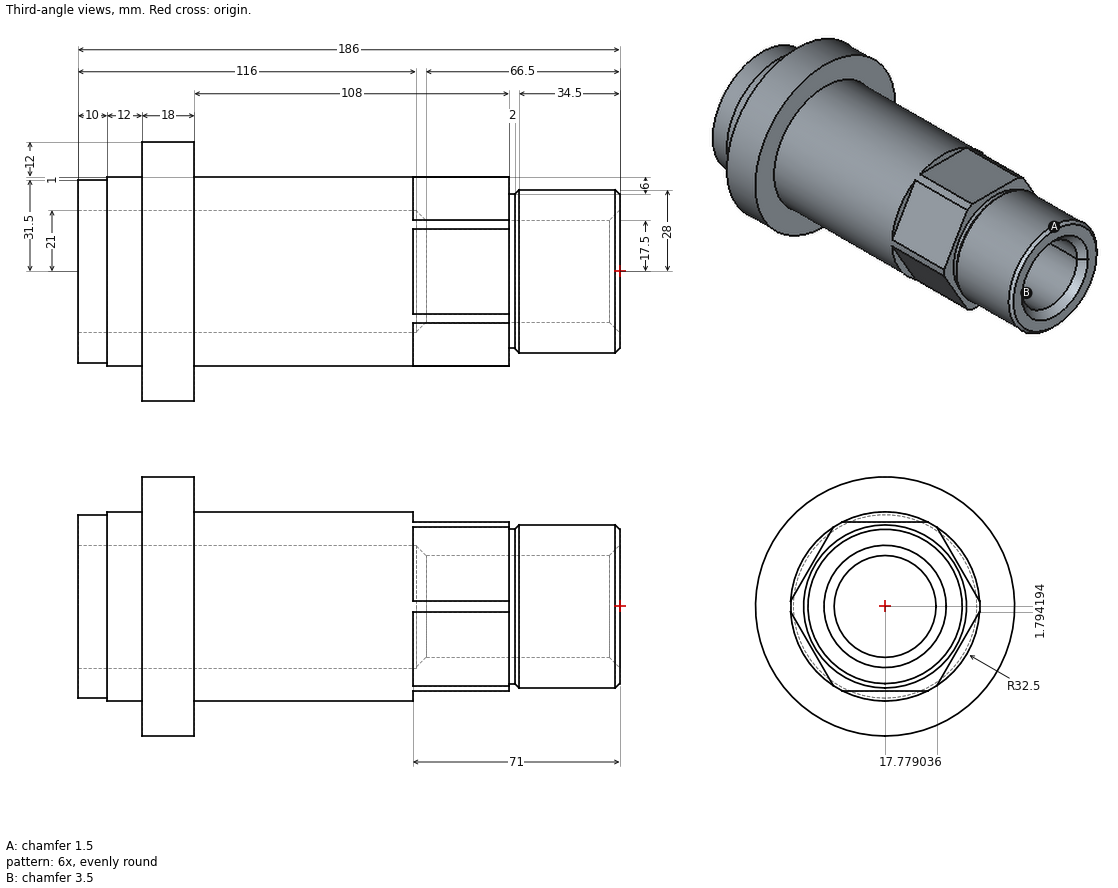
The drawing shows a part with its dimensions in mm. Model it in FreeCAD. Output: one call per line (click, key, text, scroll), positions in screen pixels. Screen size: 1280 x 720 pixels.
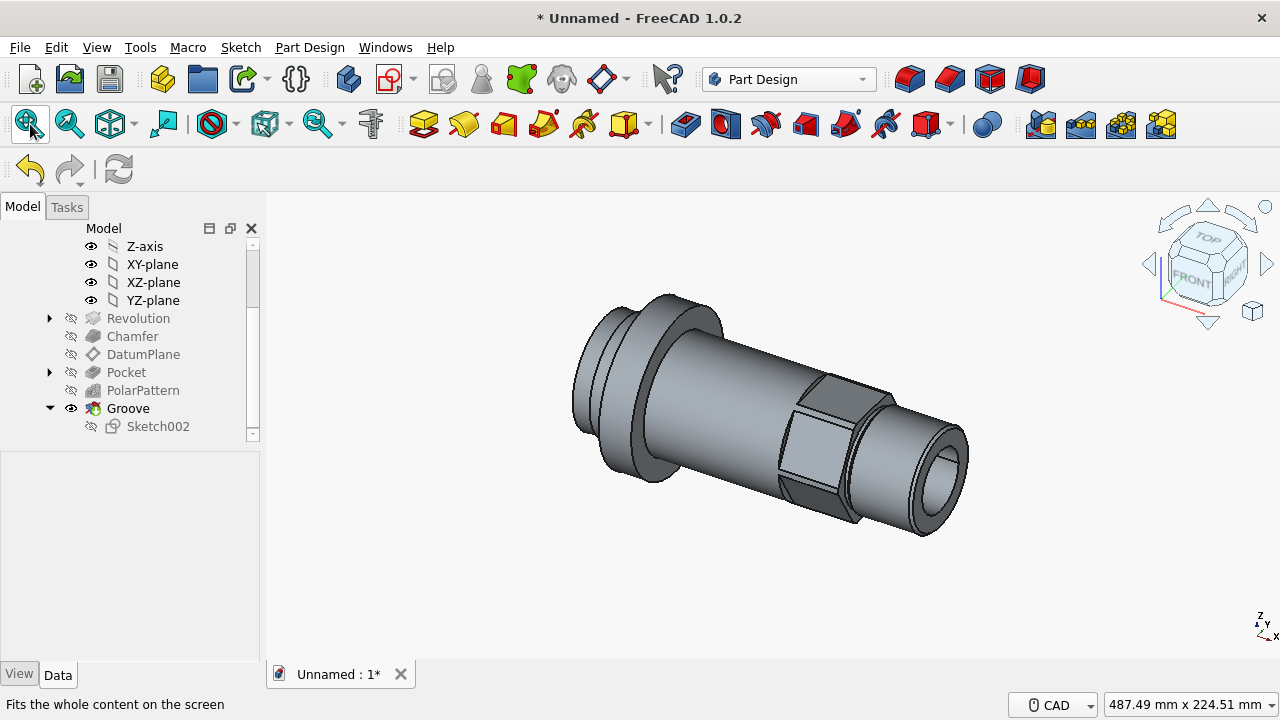
click(935, 514)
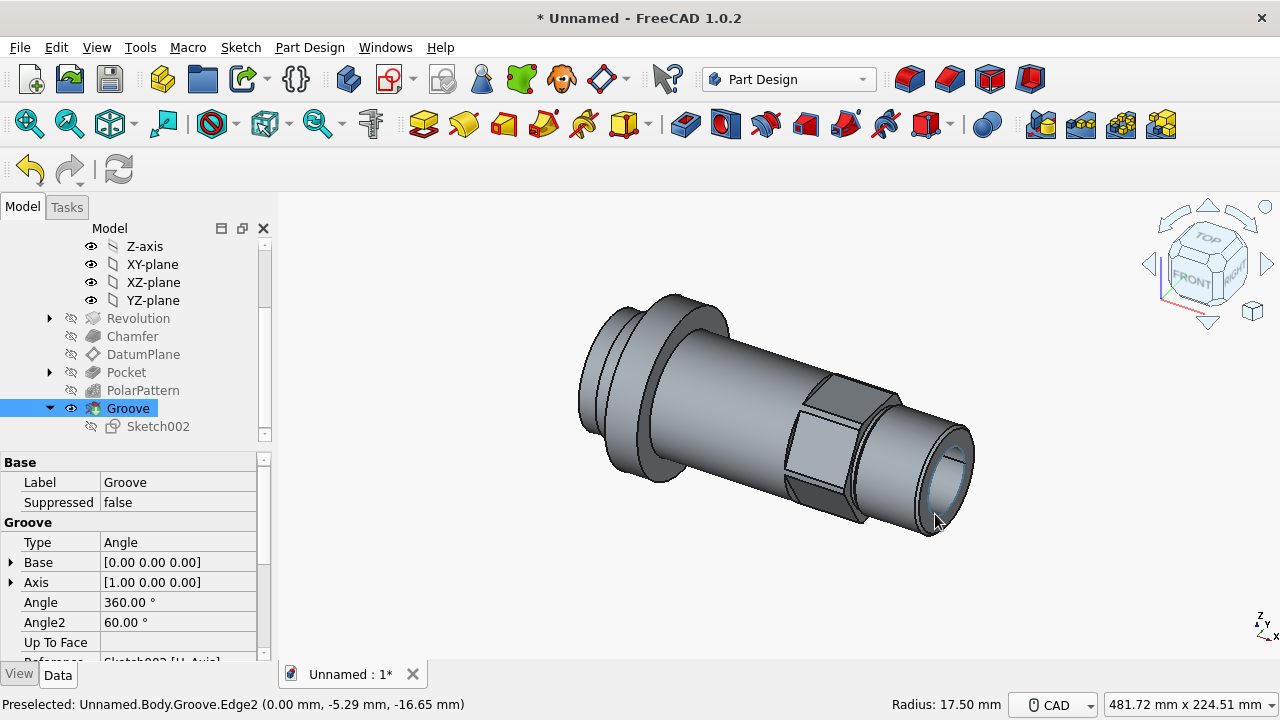
click(950, 80)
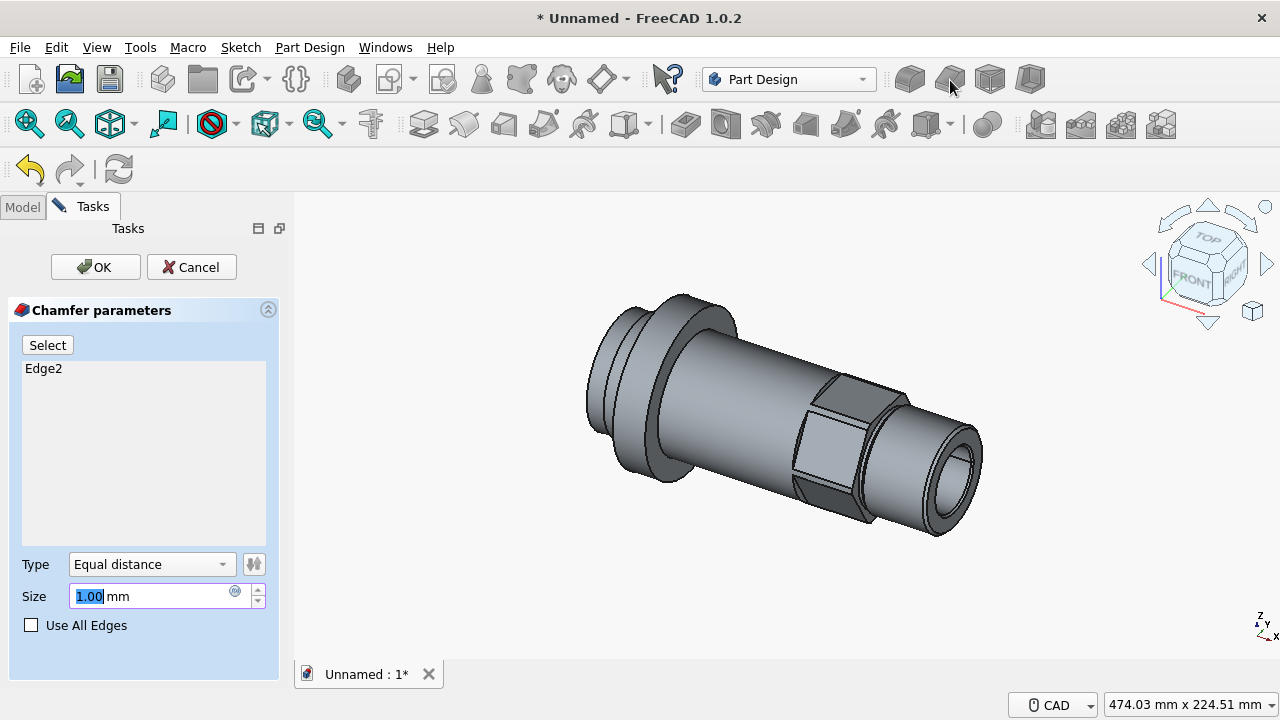
text(3.5)
key(Tab)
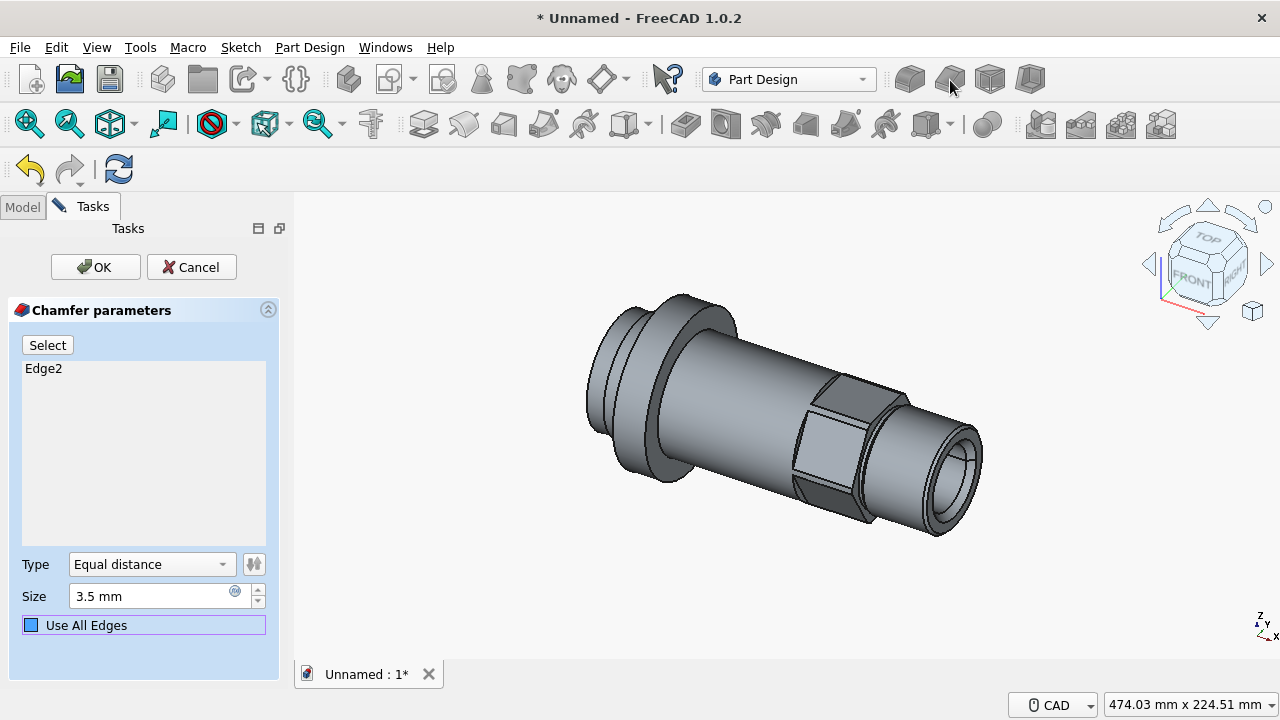
click(96, 267)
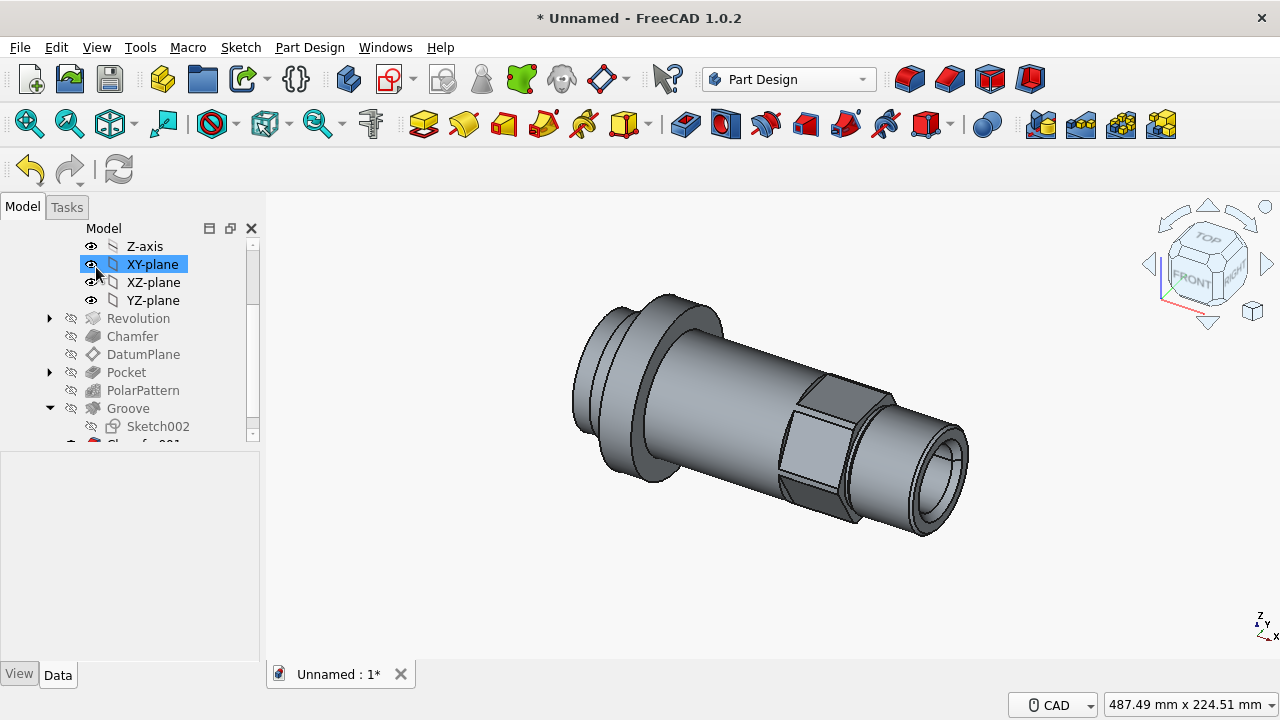
key(0)